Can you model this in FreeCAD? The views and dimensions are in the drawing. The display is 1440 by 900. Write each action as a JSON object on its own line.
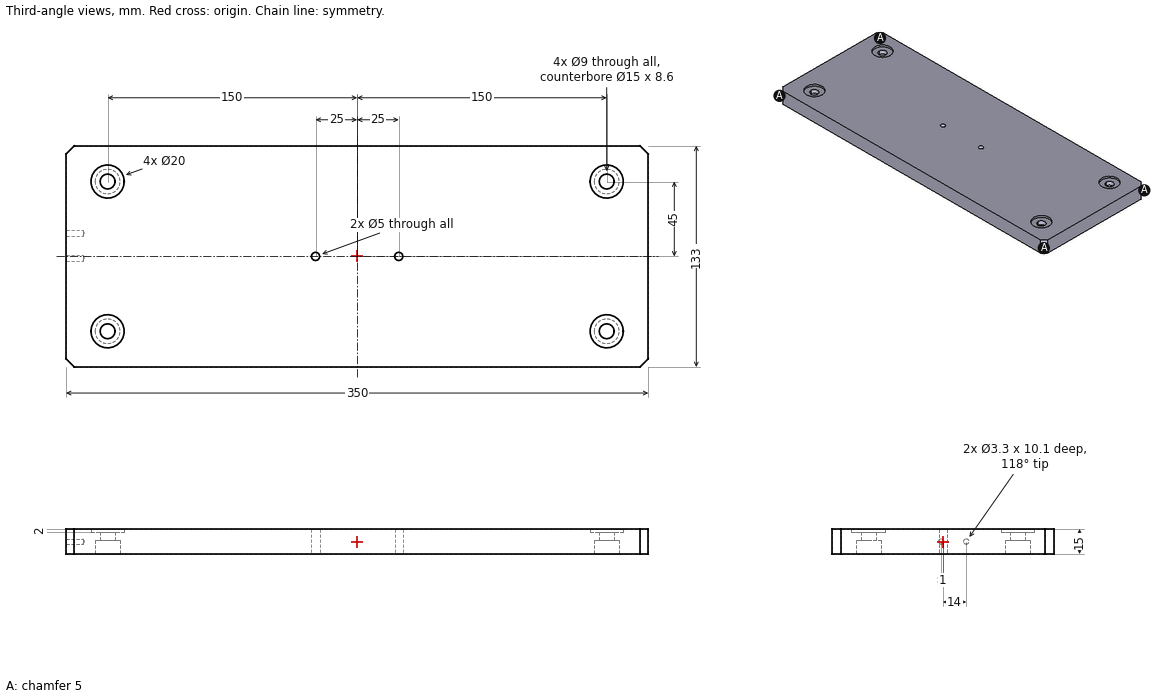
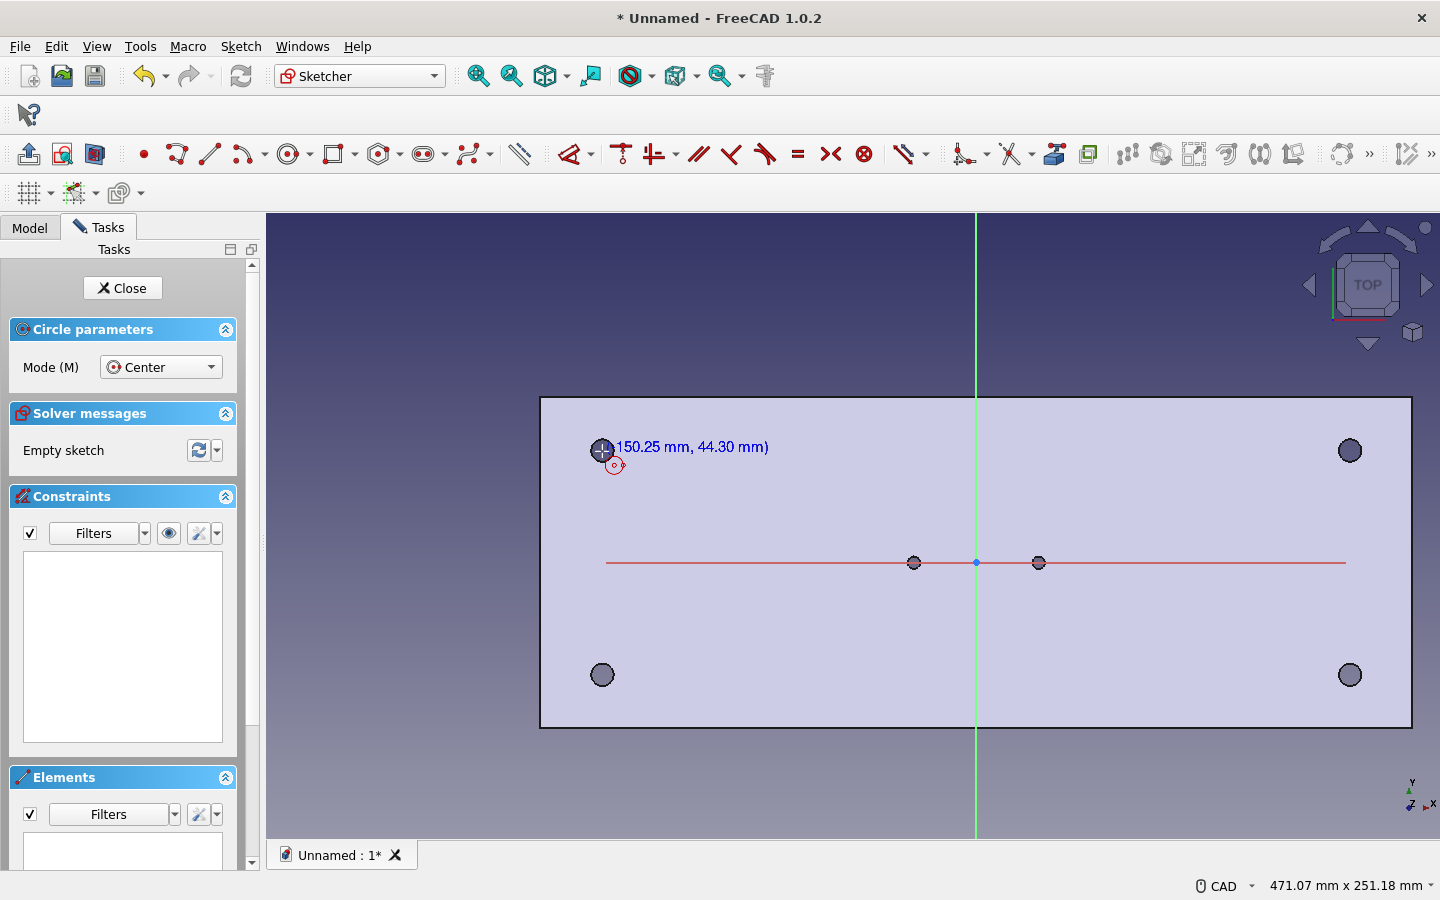
{"action": "left_click", "coordinate": [602, 451]}
{"action": "mouse_move", "coordinate": [620, 433]}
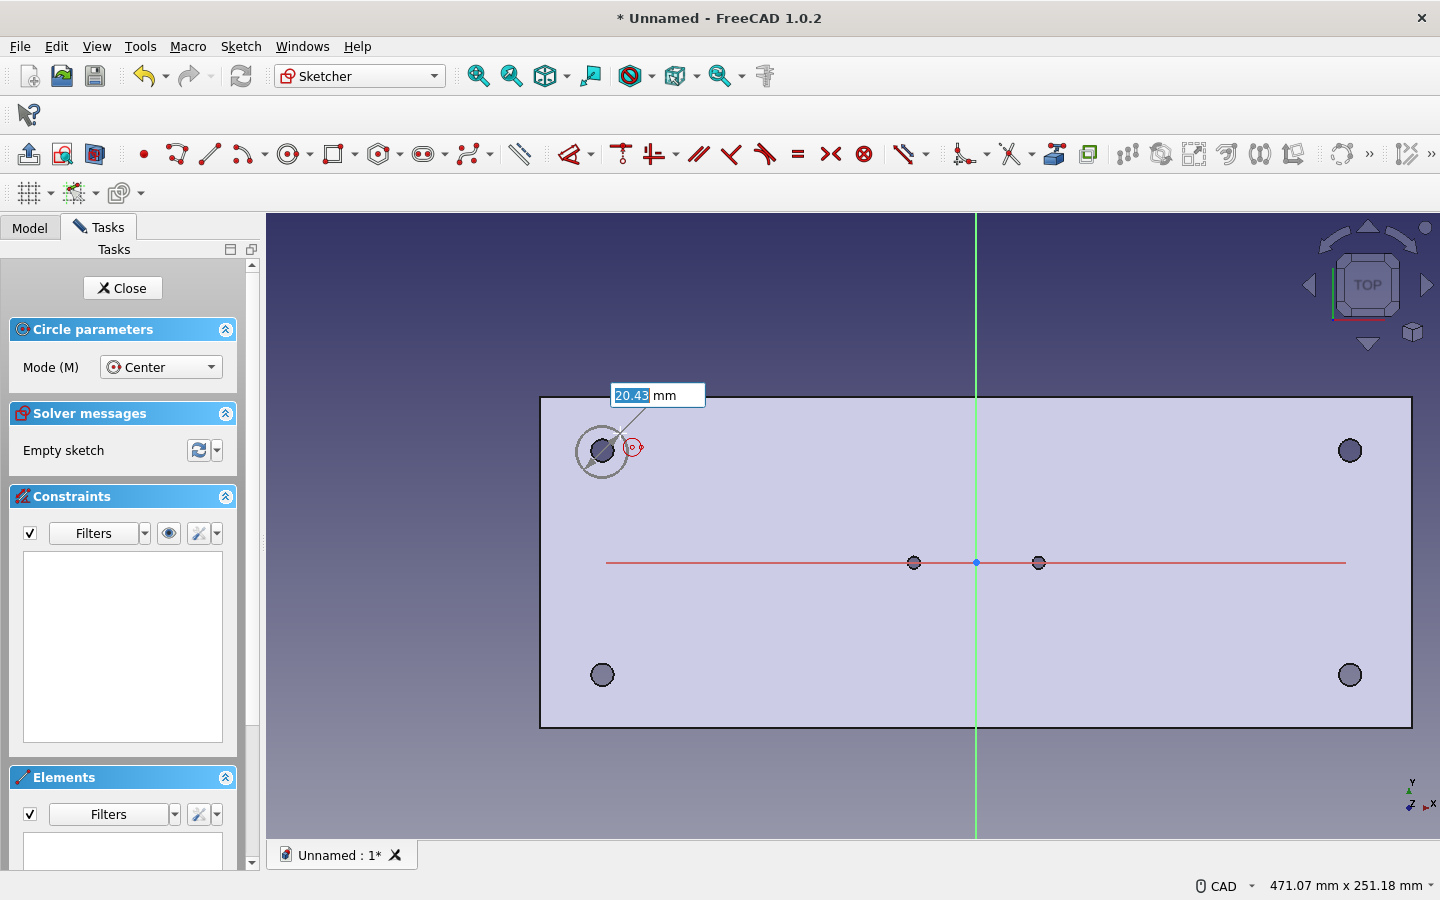
{"action": "type", "text": "20"}
{"action": "key", "text": "Return"}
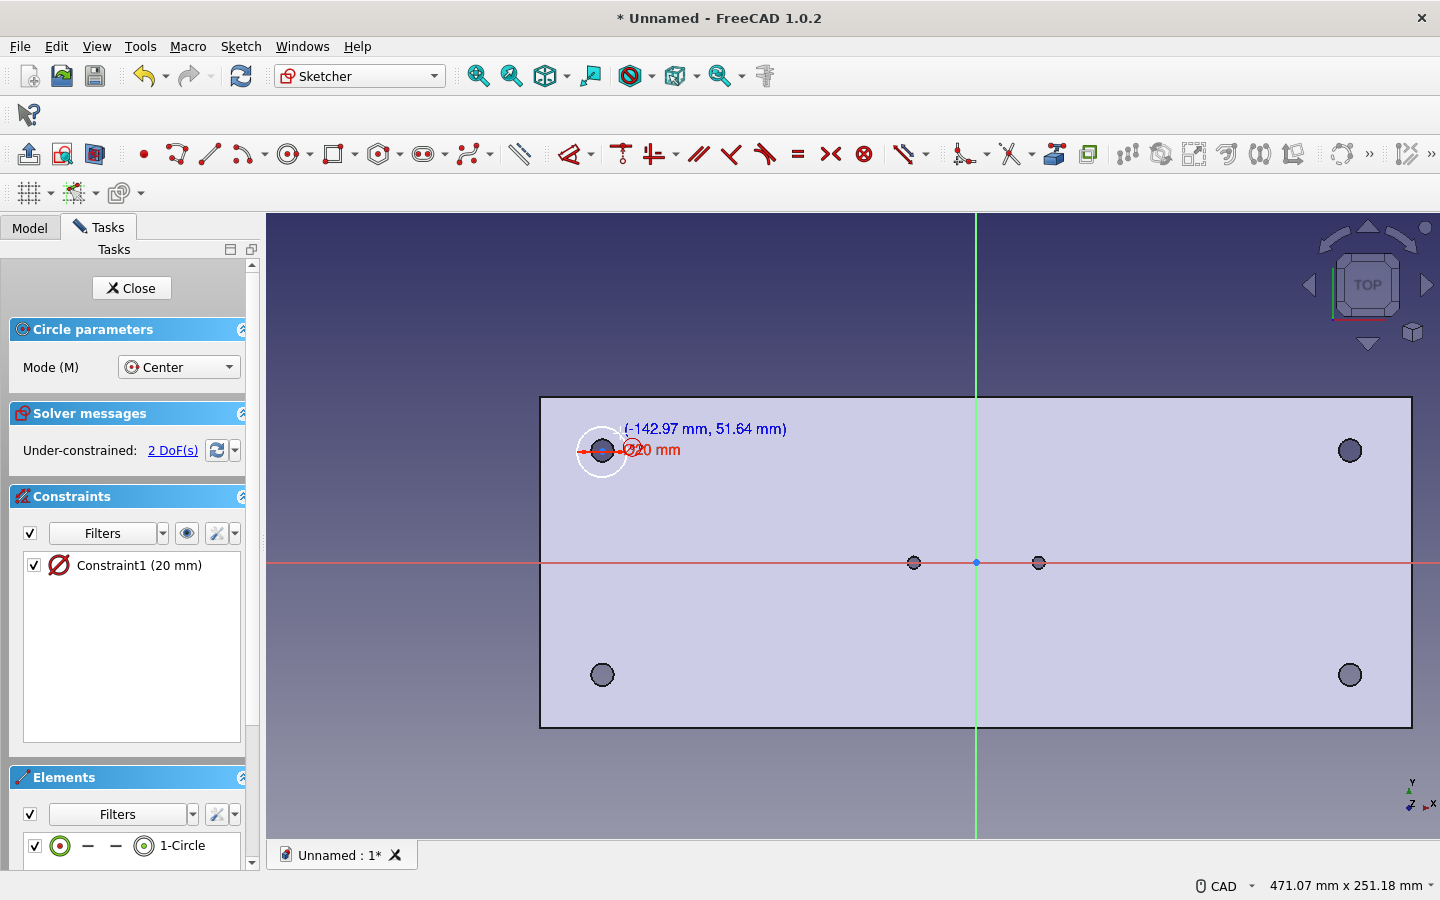
{"action": "left_click", "coordinate": [602, 675]}
{"action": "mouse_move", "coordinate": [620, 657]}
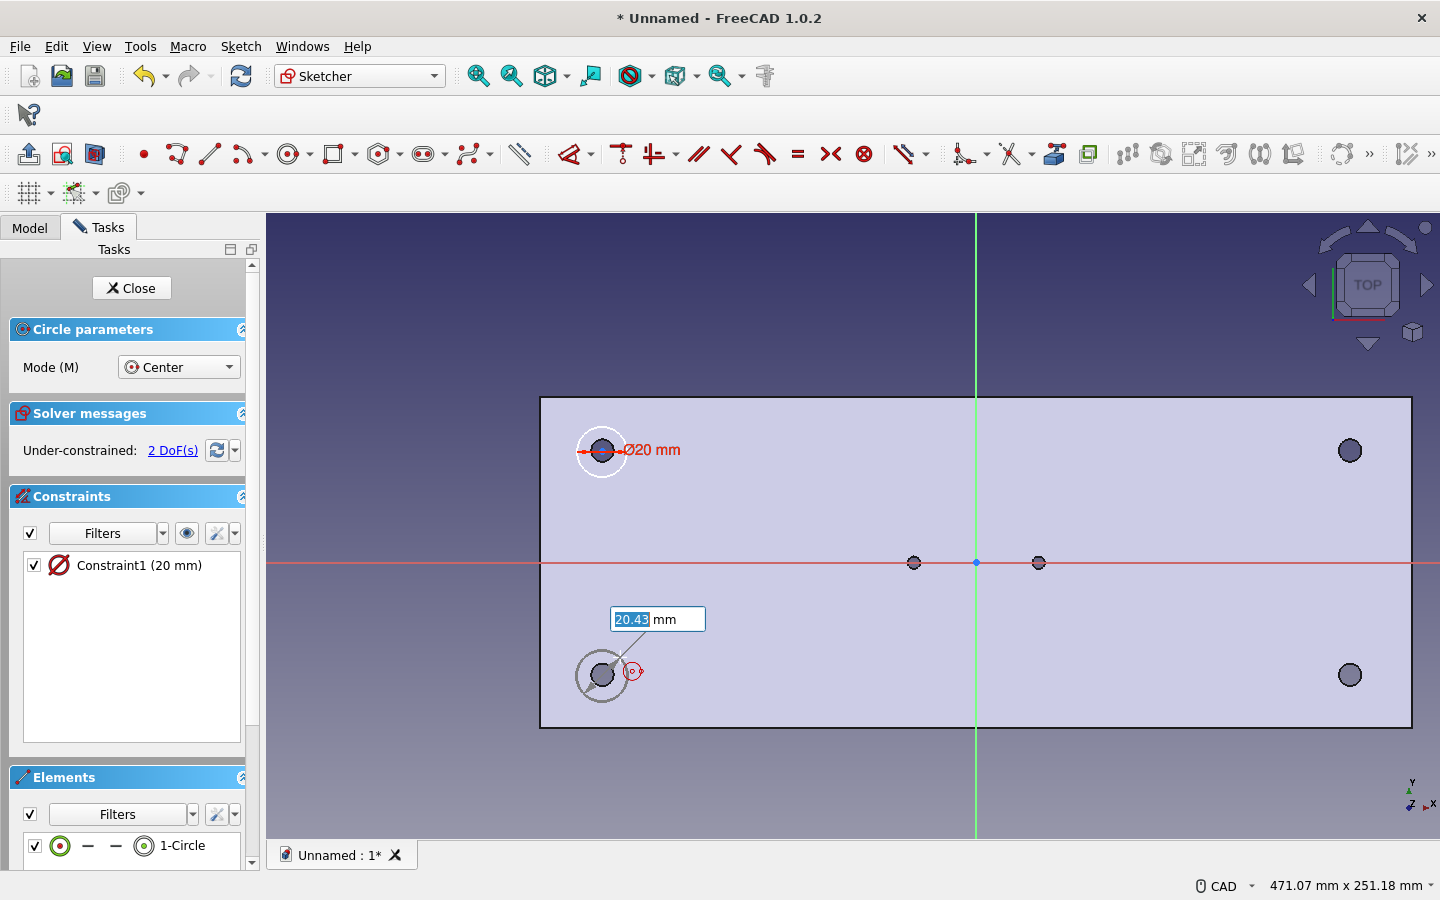
{"action": "type", "text": "20"}
{"action": "key", "text": "Return"}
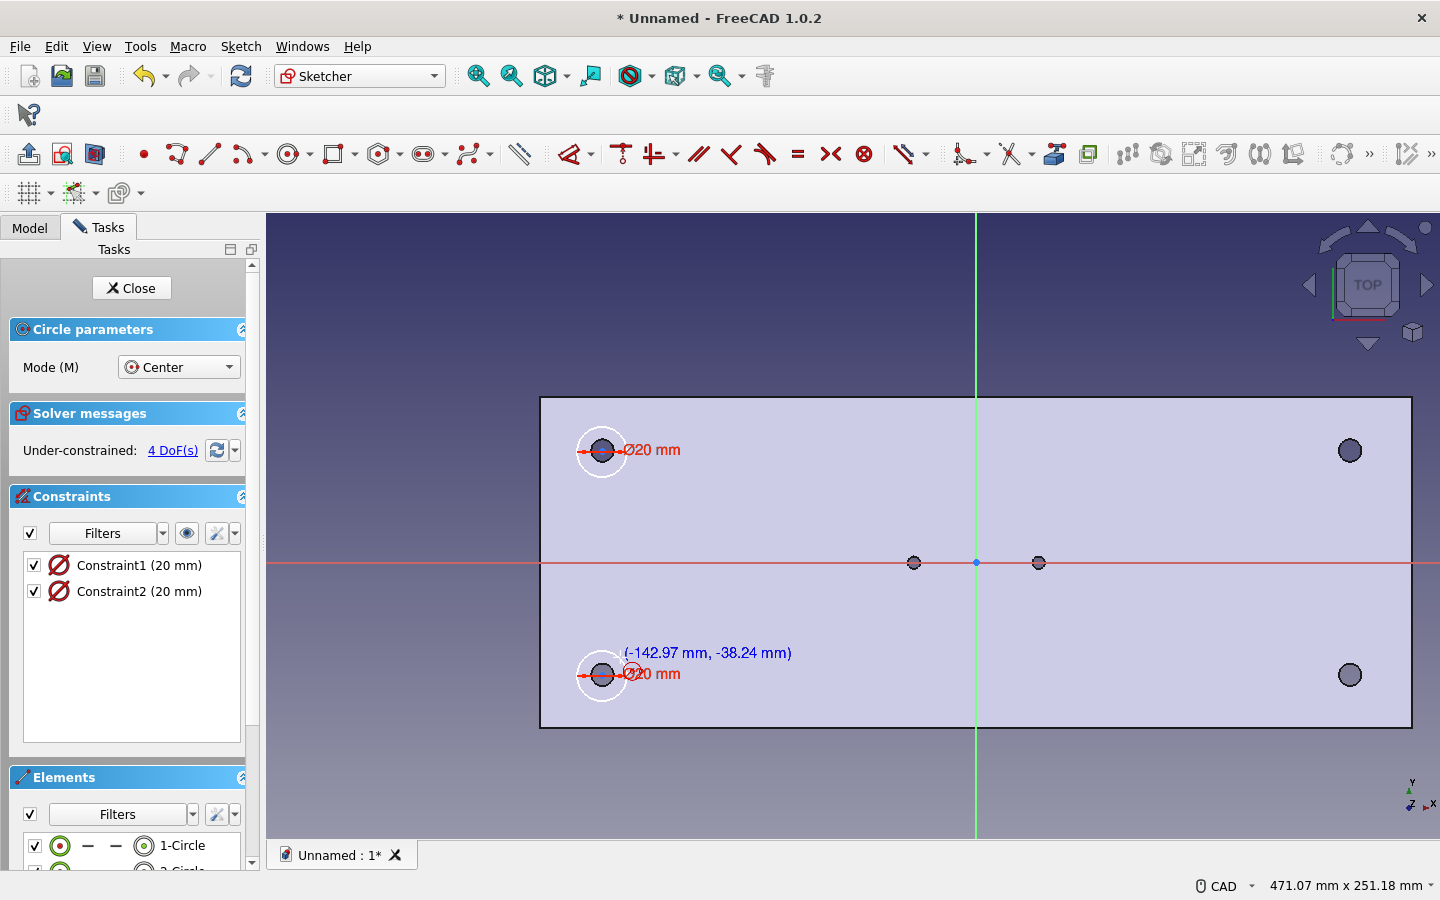
{"action": "scroll", "coordinate": [294, 360], "scroll_direction": "down", "scroll_amount": 1}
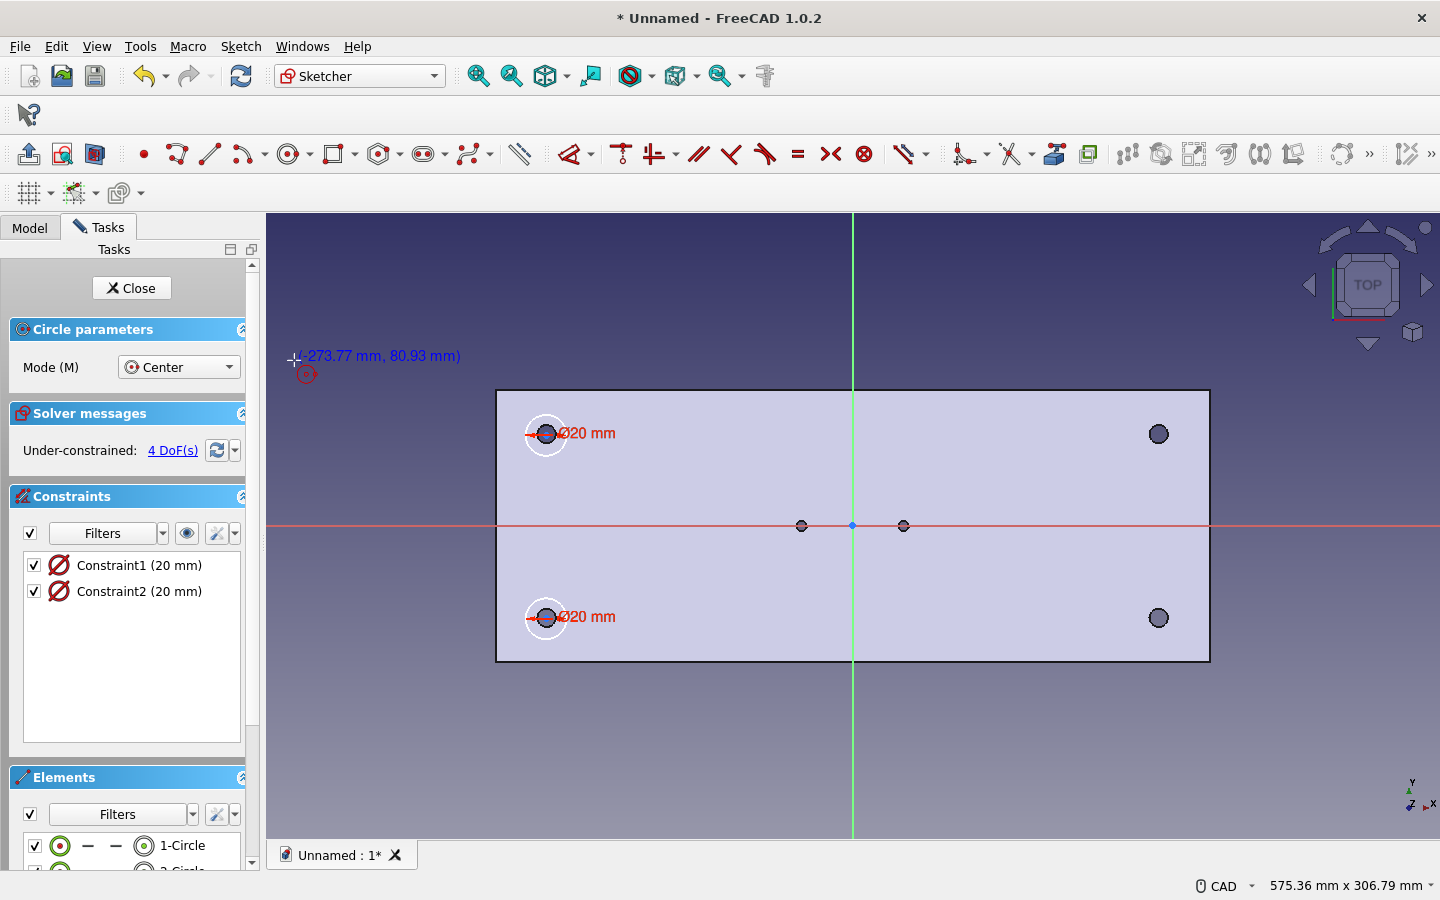
{"action": "left_click", "coordinate": [1159, 618]}
{"action": "mouse_move", "coordinate": [1173, 603]}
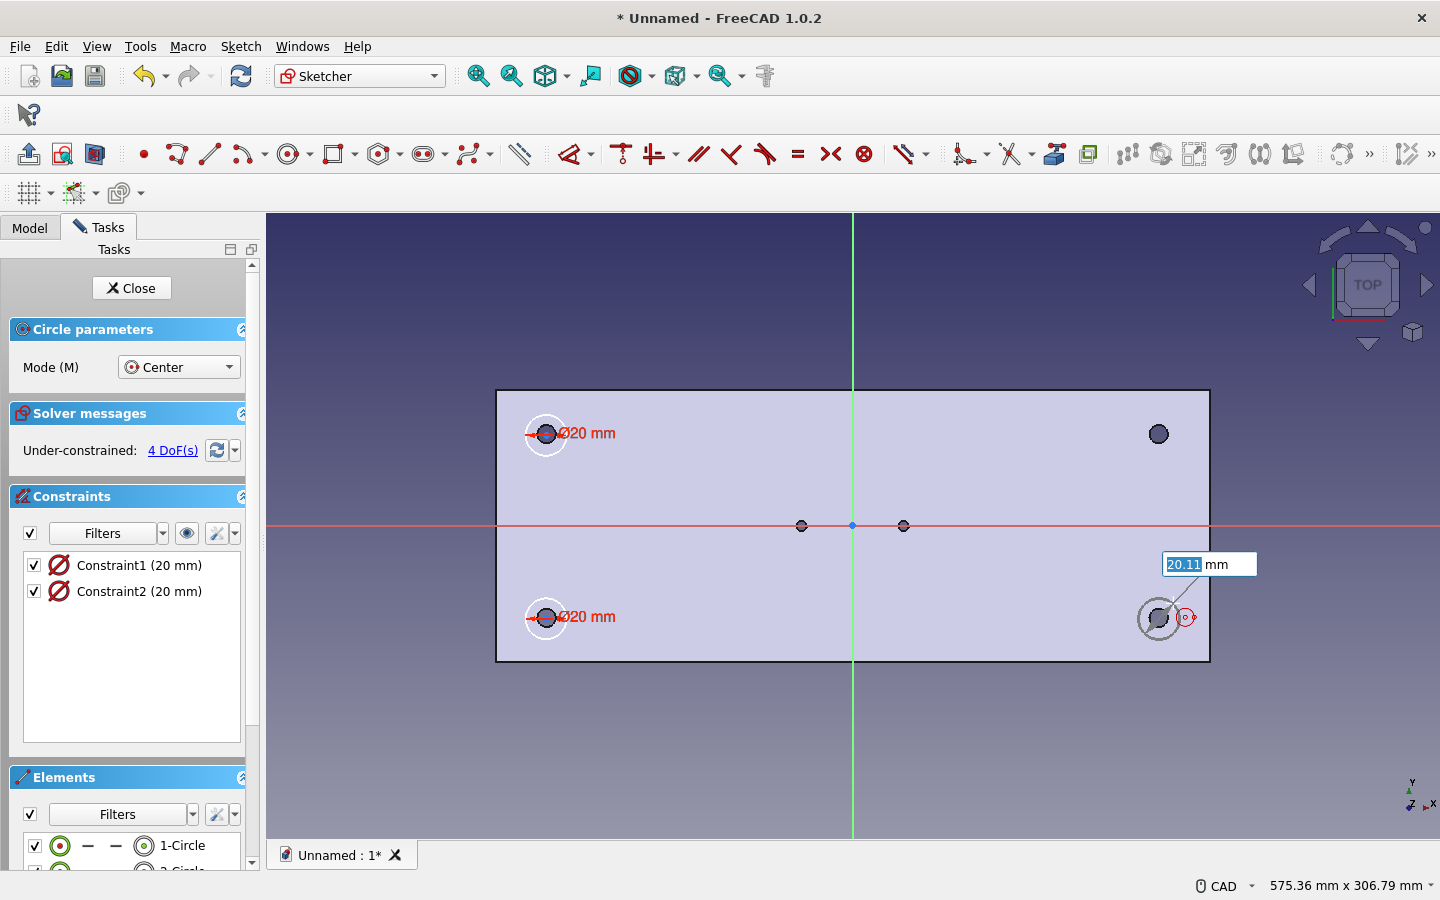
{"action": "type", "text": "20"}
{"action": "key", "text": "Return"}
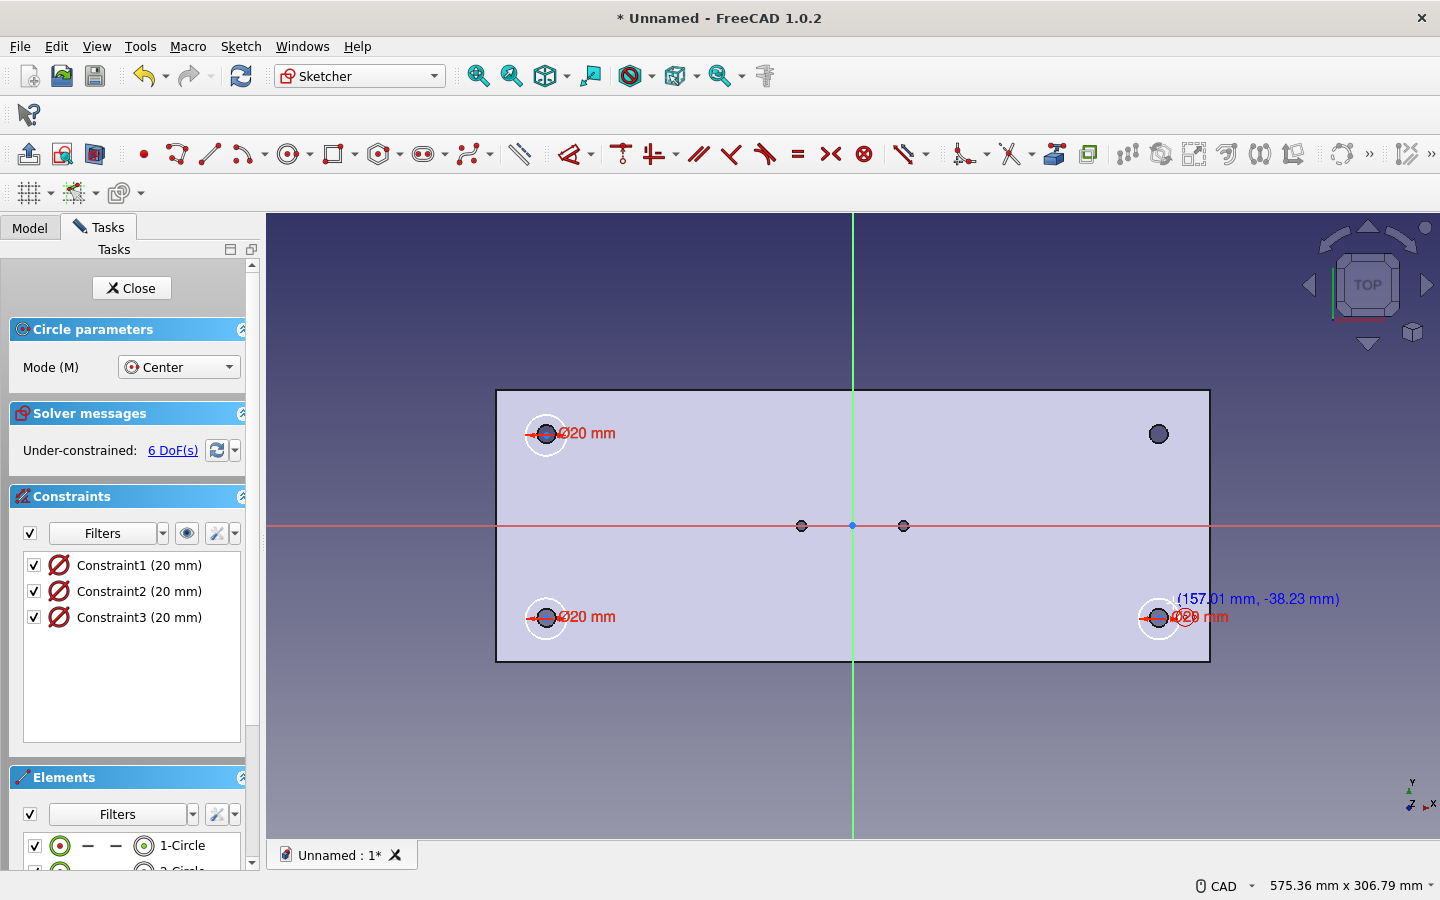
{"action": "left_click", "coordinate": [1159, 434]}
{"action": "mouse_move", "coordinate": [1173, 420]}